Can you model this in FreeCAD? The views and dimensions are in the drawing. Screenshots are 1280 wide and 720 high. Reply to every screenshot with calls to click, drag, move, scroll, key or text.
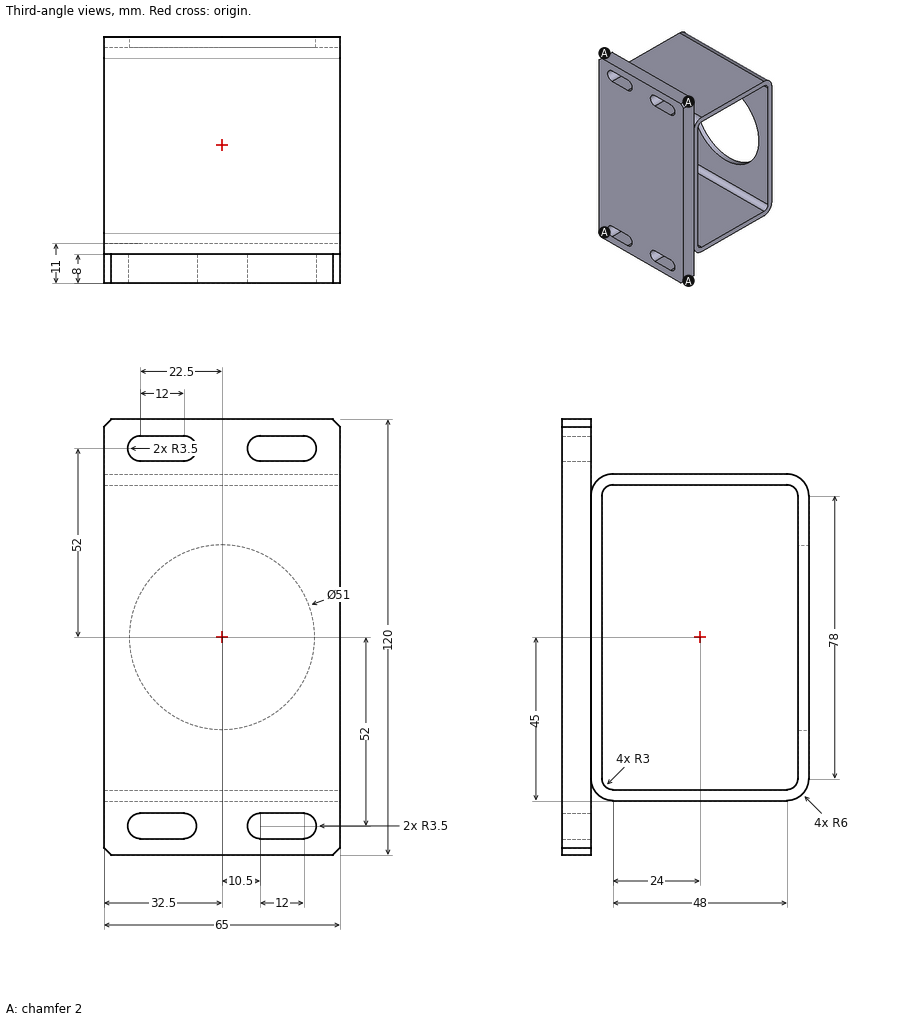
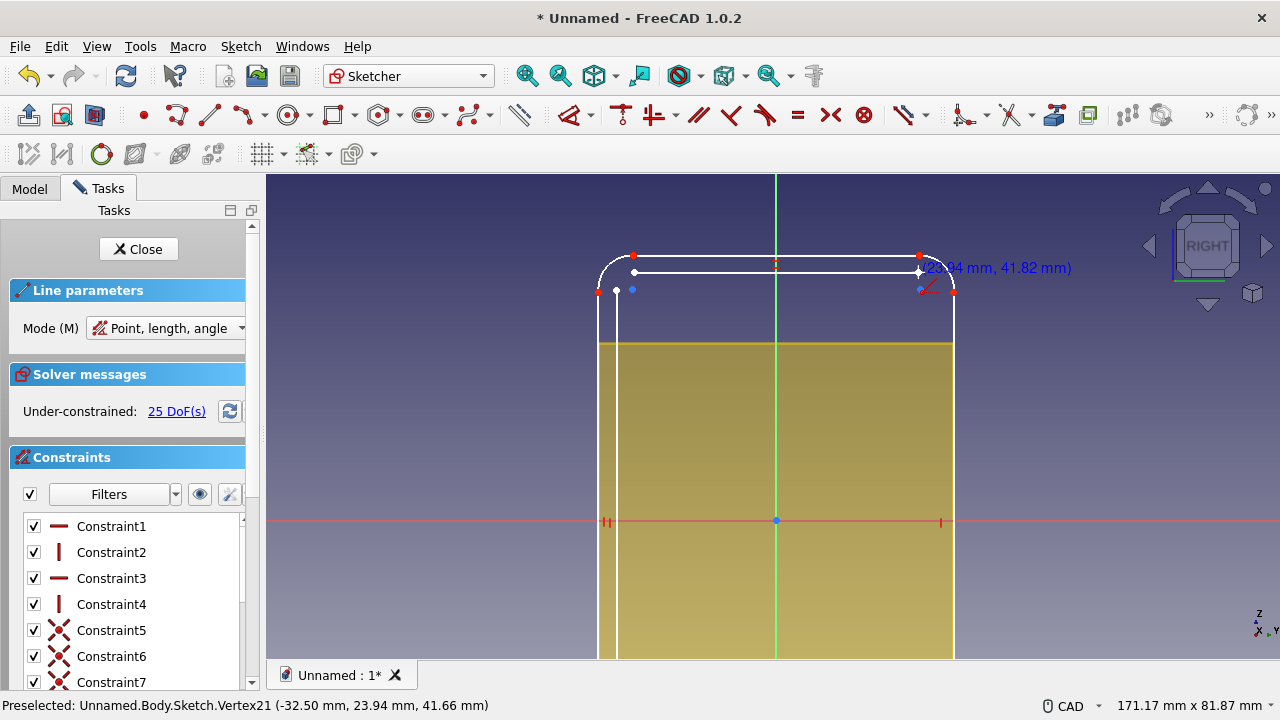
click(936, 290)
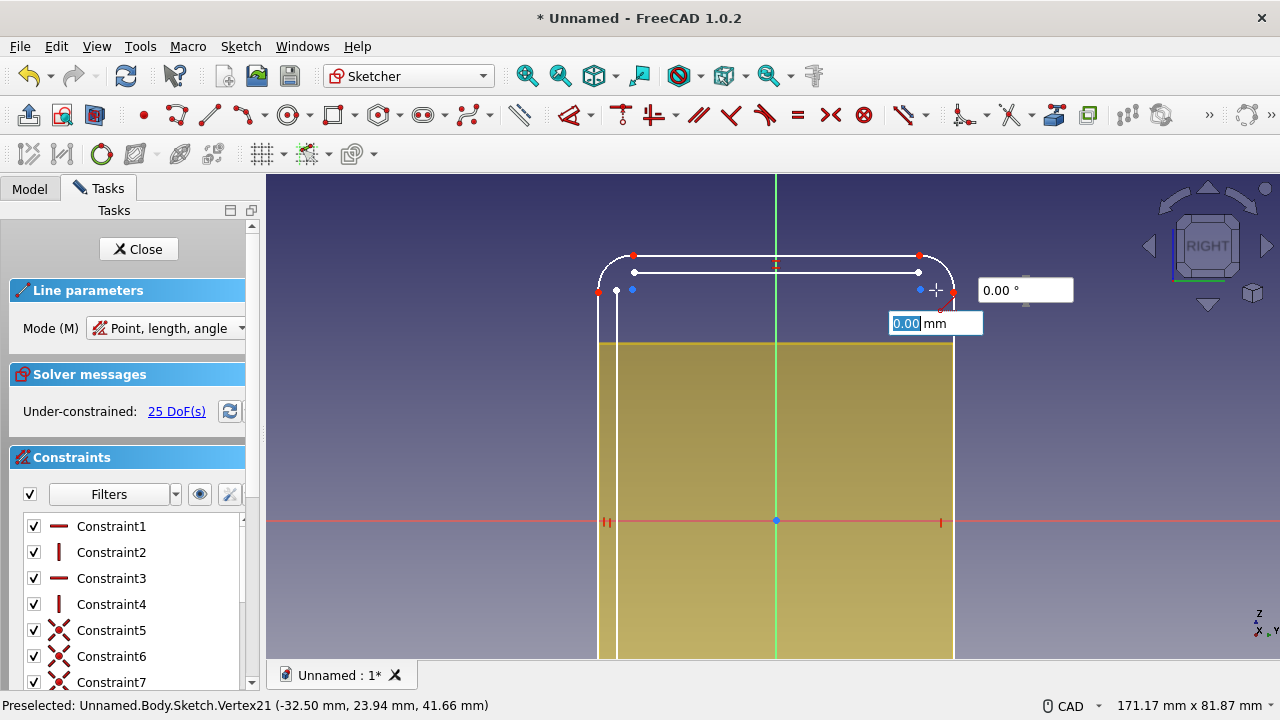
scroll(617, 290, down, 3)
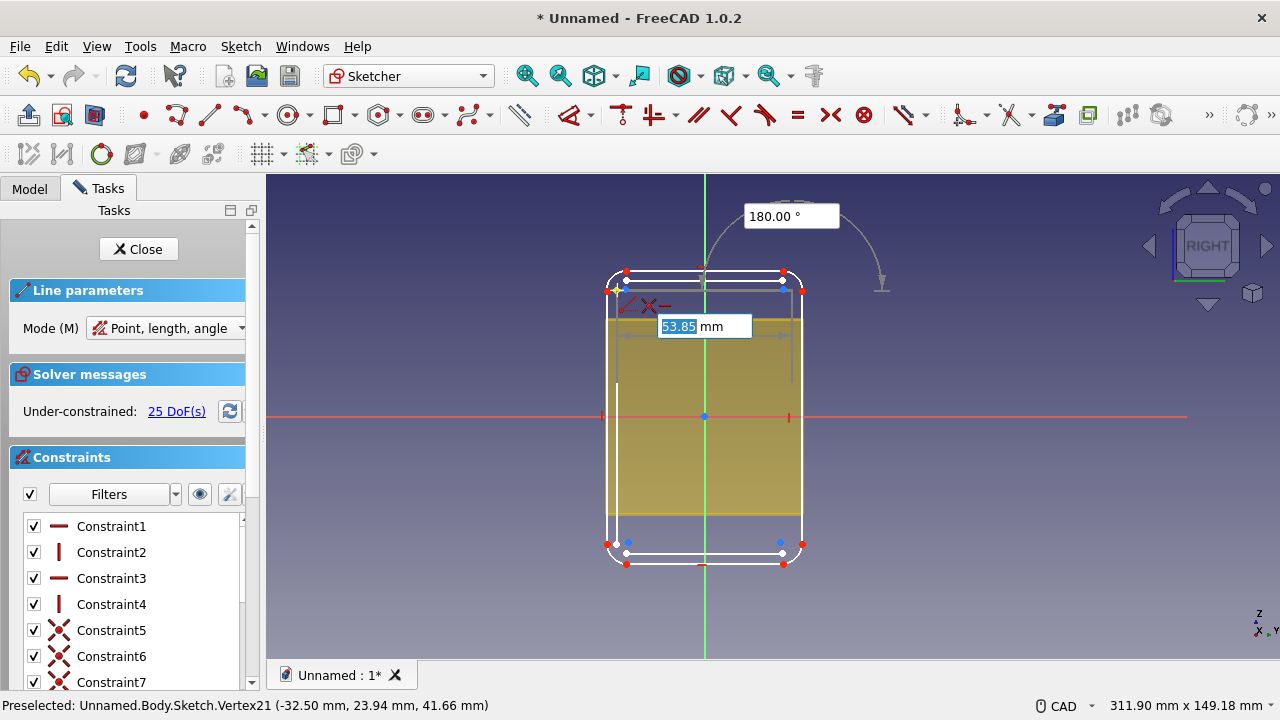
scroll(792, 544, up, 3)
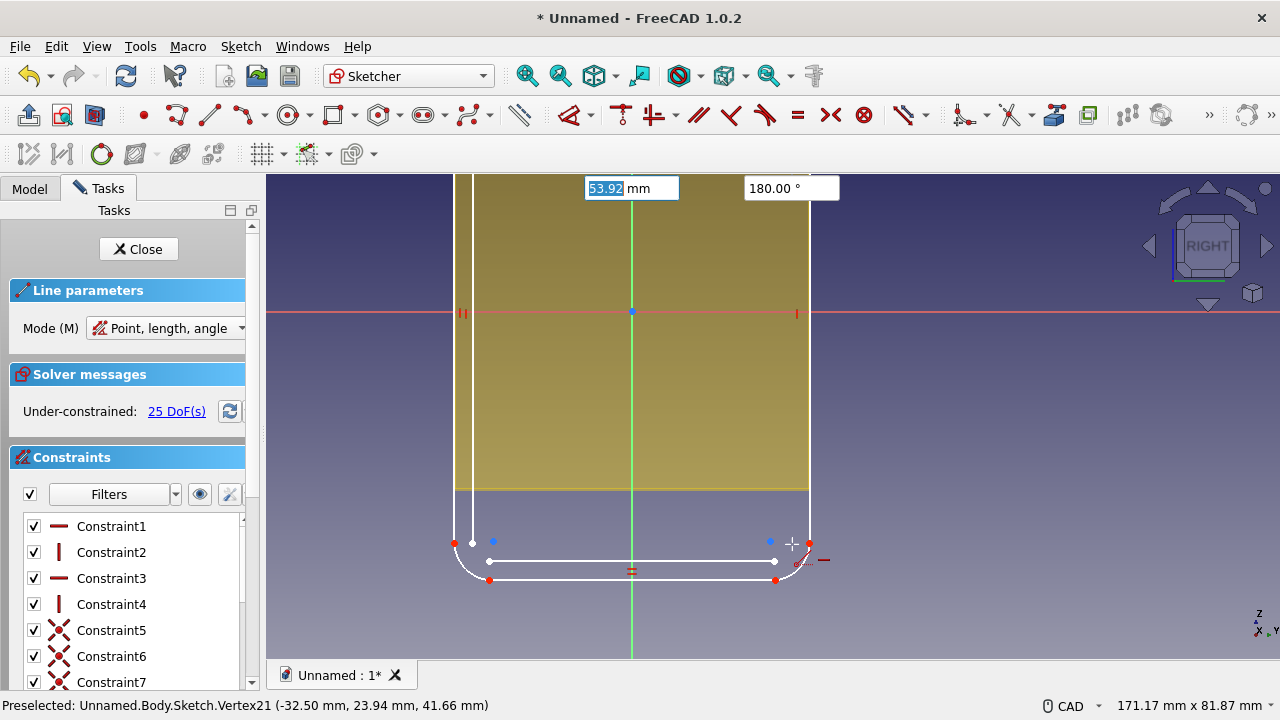
click(792, 543)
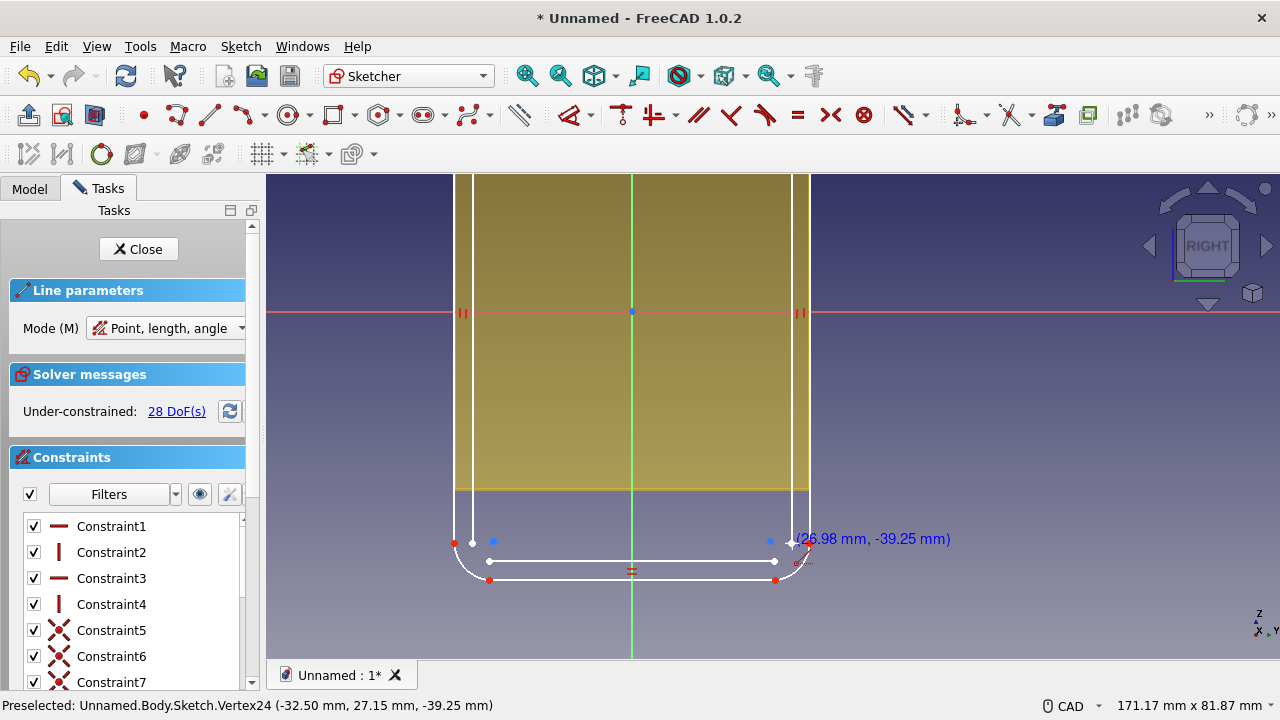
click(242, 116)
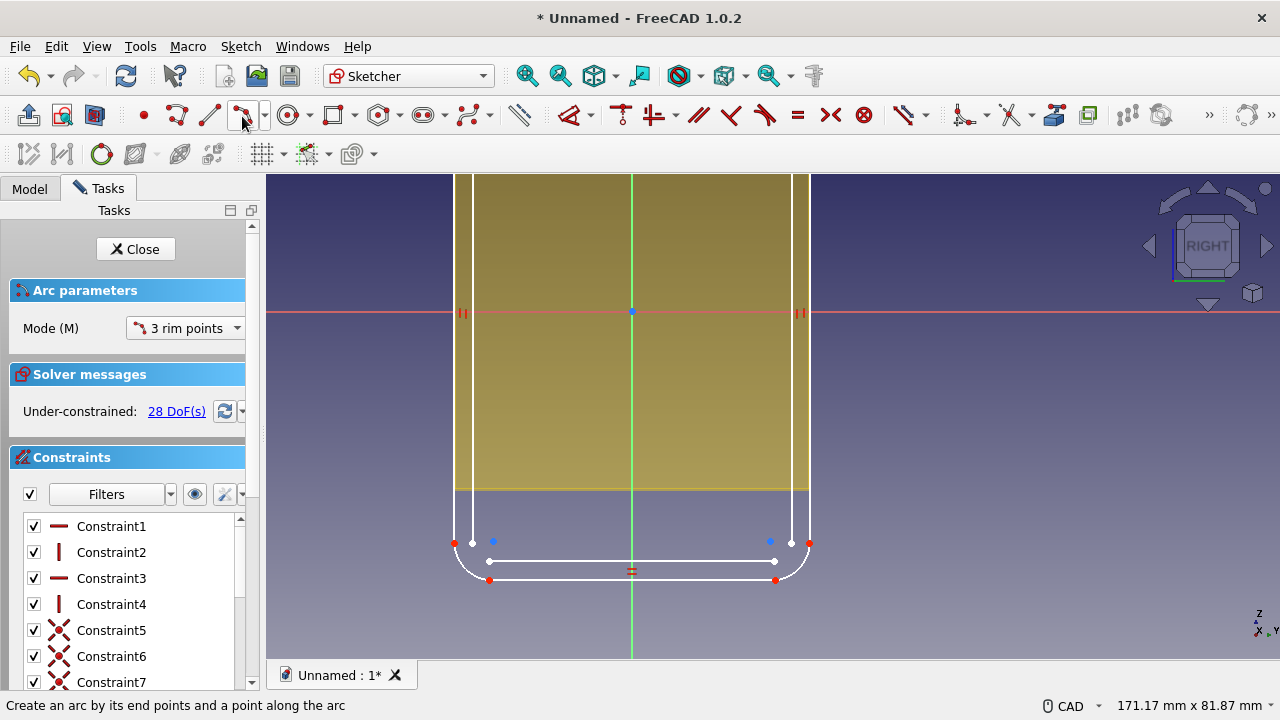
click(490, 561)
click(473, 543)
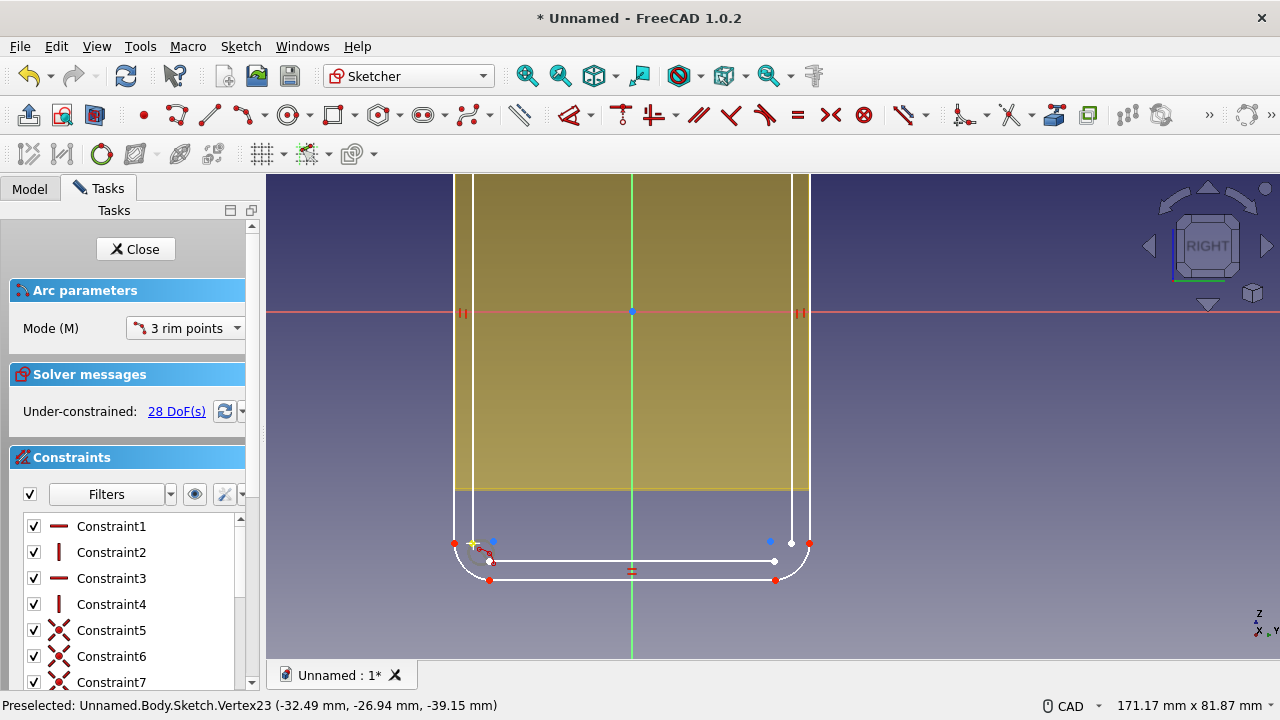
scroll(477, 555, up, 6)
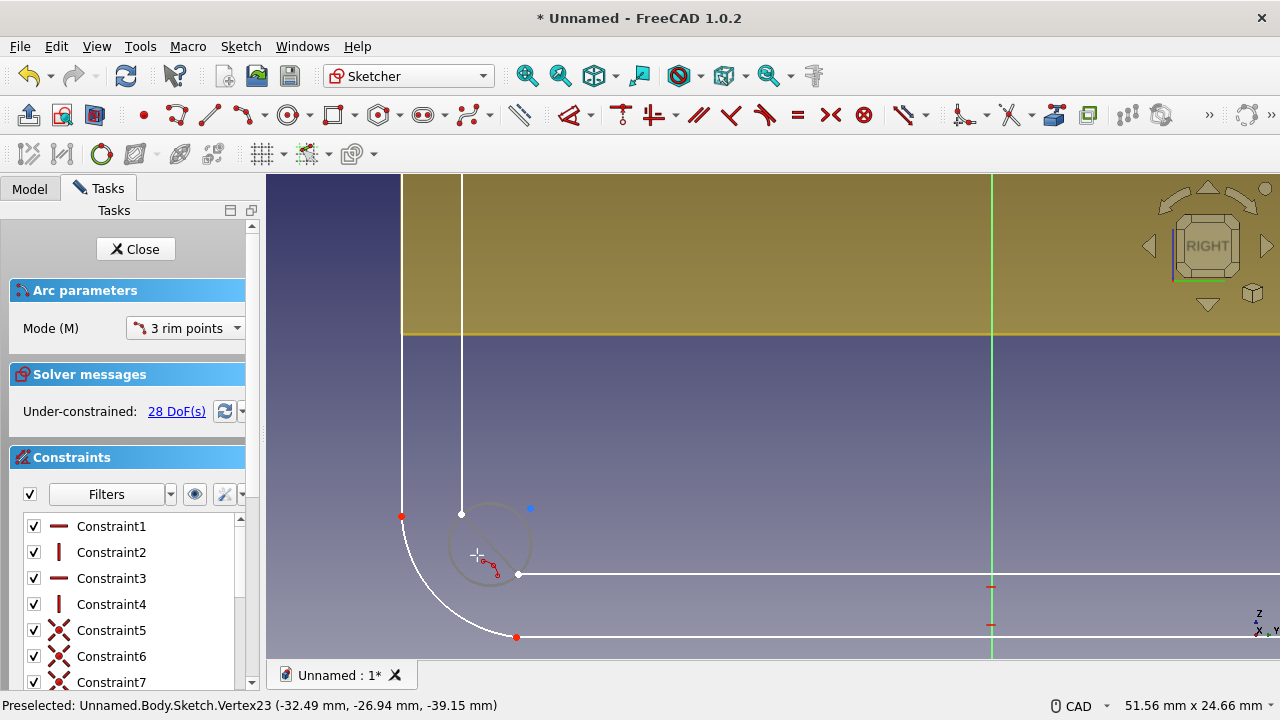
click(478, 553)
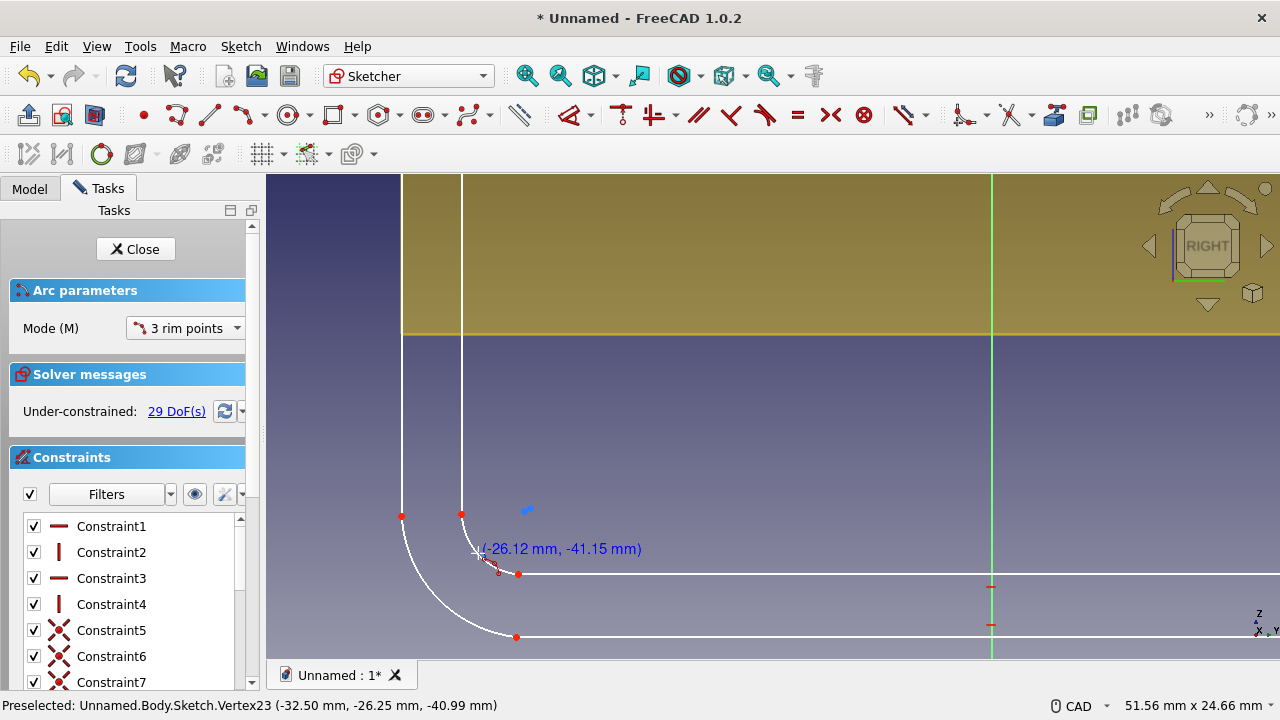
scroll(648, 550, down, 9)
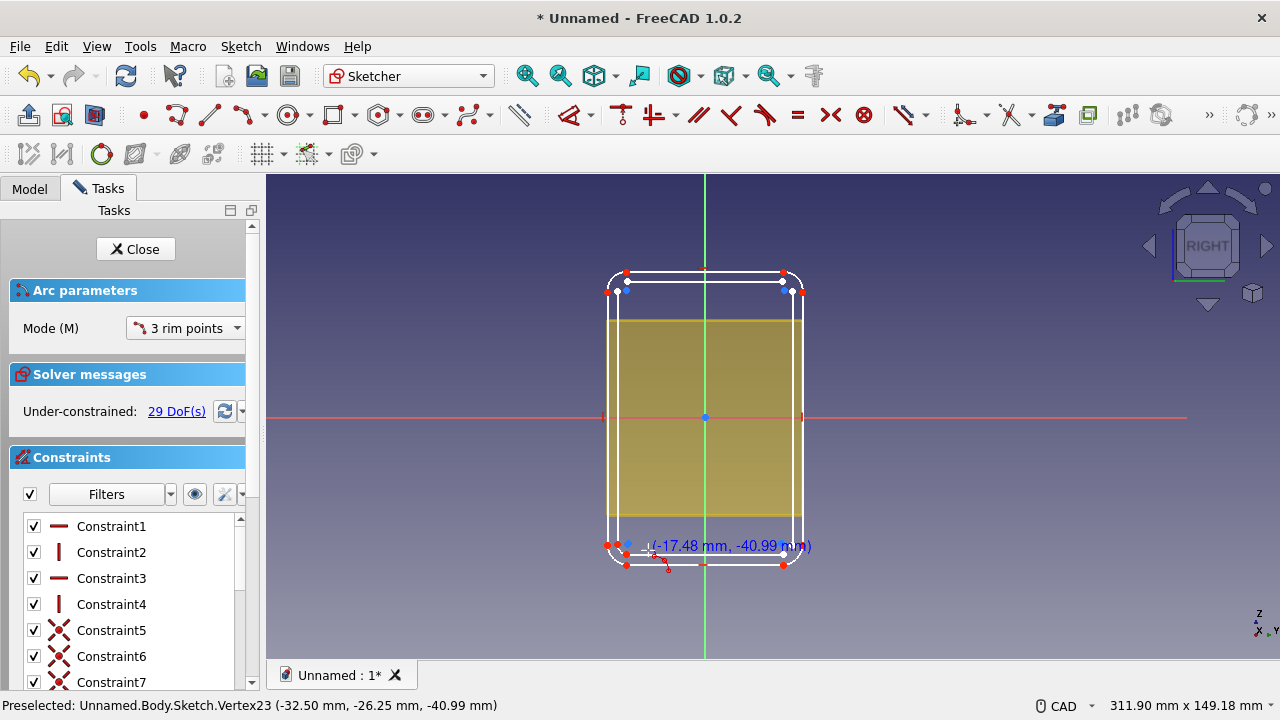
scroll(617, 291, up, 3)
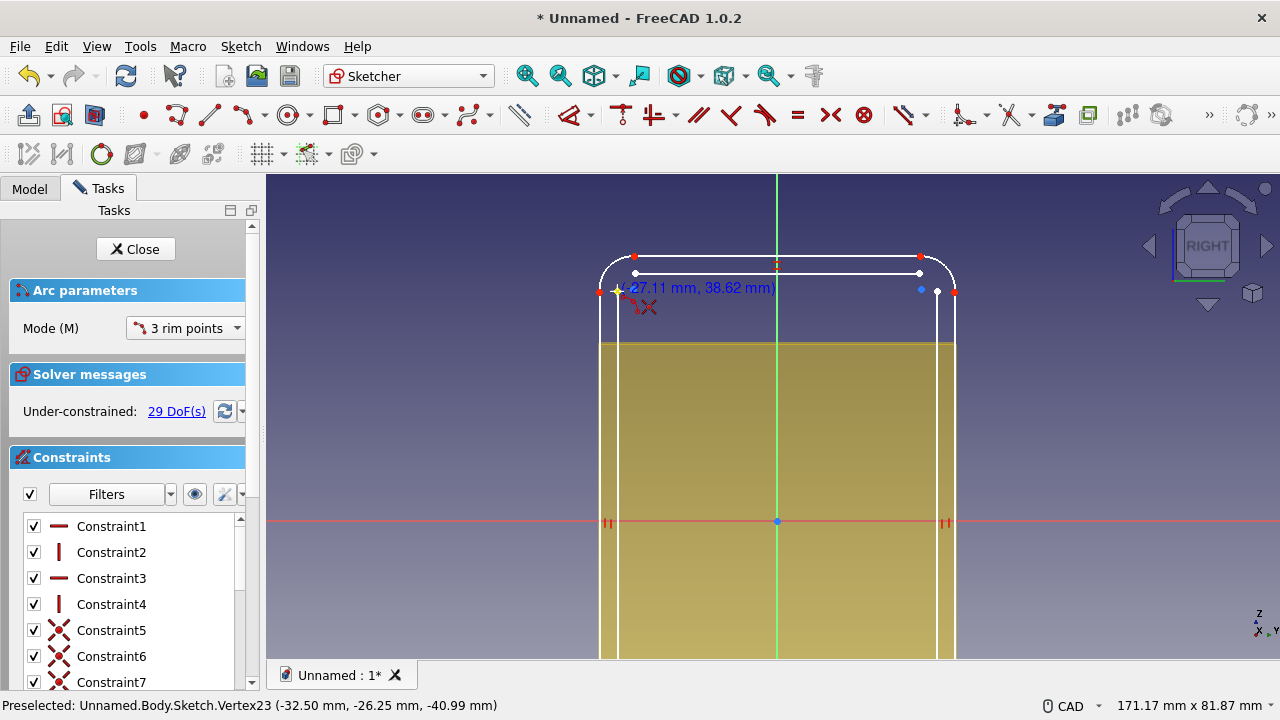
click(618, 292)
click(635, 274)